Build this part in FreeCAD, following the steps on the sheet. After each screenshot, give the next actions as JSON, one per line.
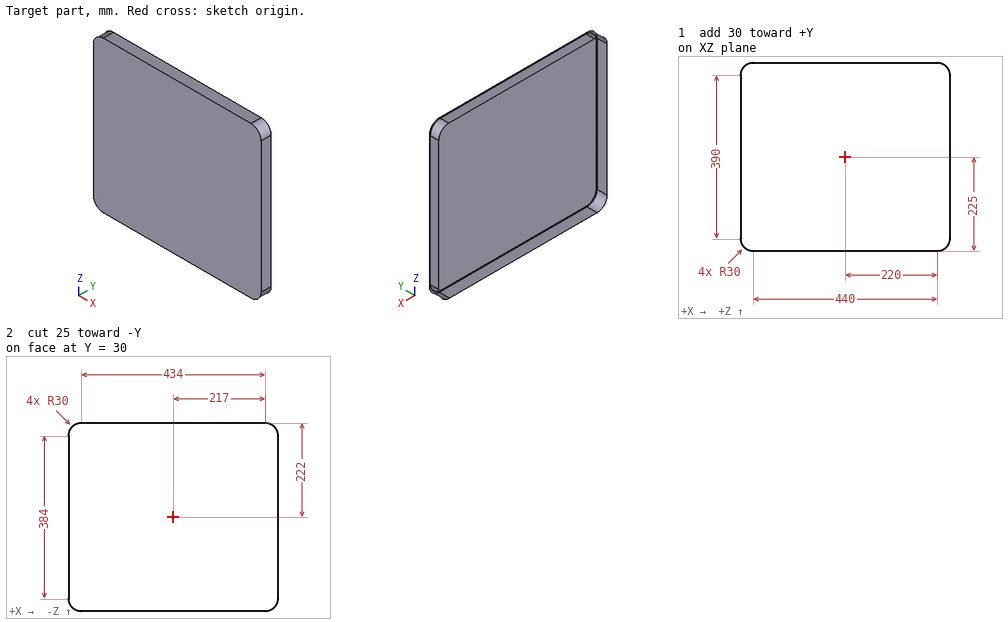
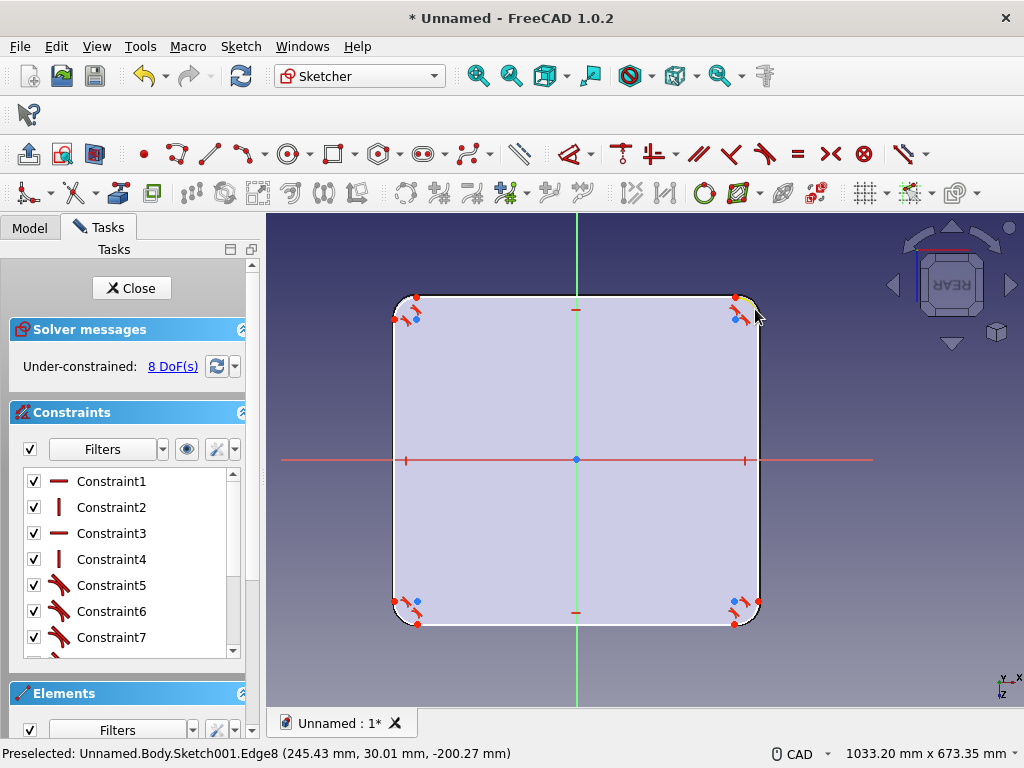
{"action": "scroll", "coordinate": [407, 300], "scroll_direction": "up", "scroll_amount": 2}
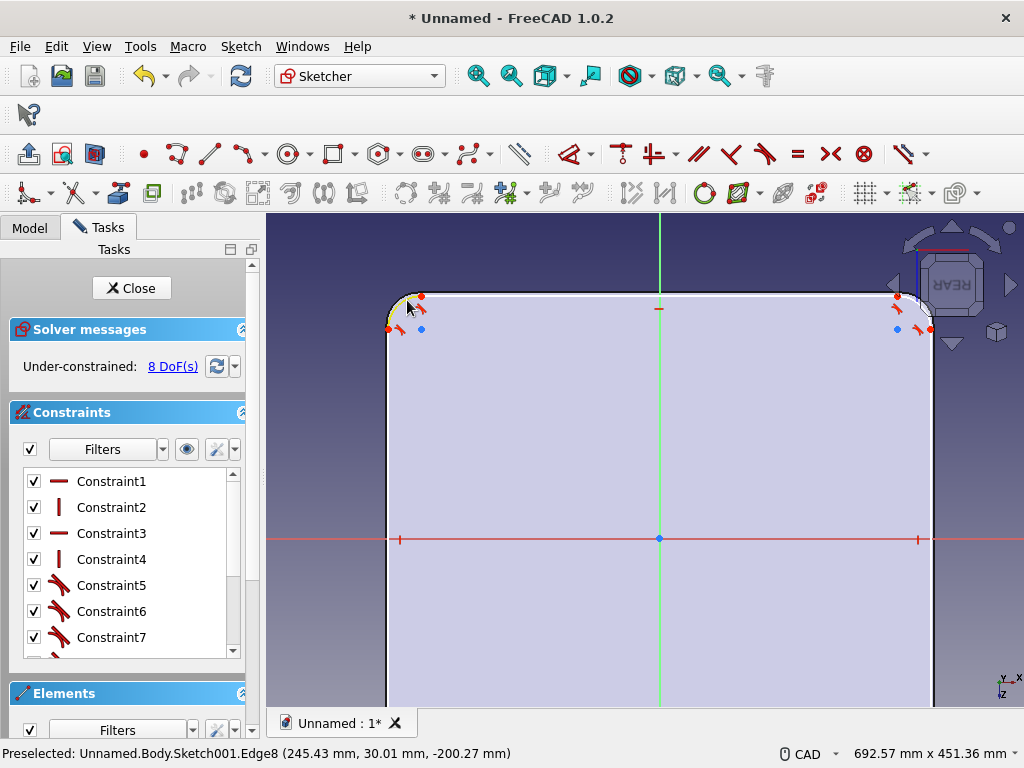
{"action": "left_click", "coordinate": [406, 300]}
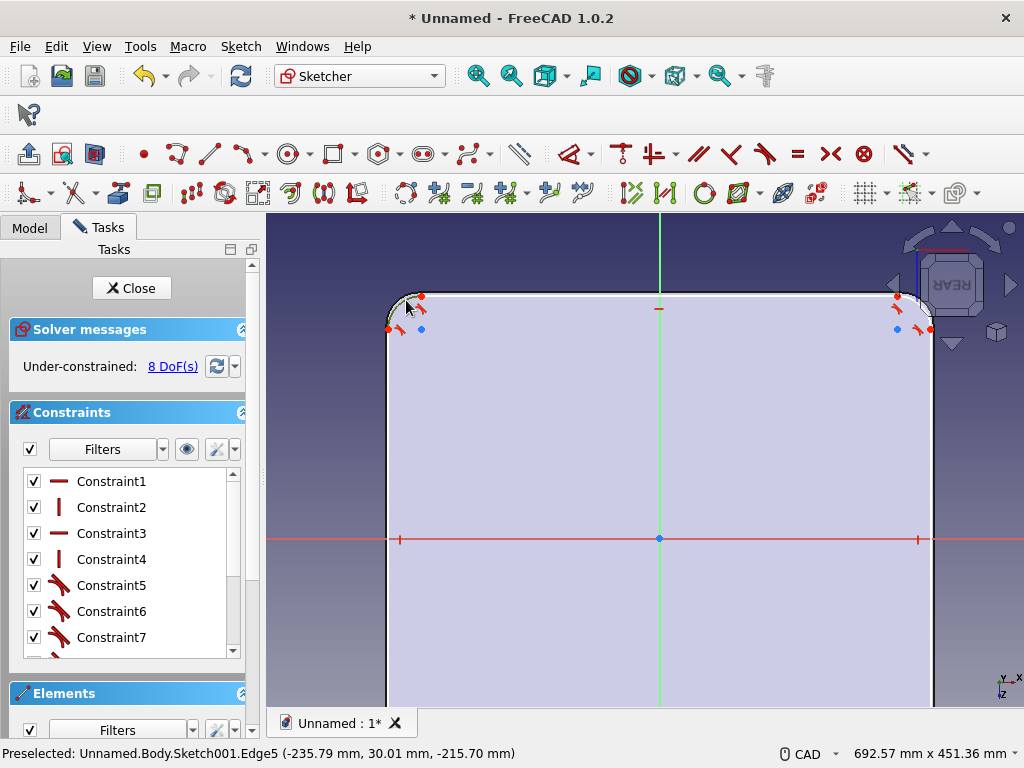
{"action": "scroll", "coordinate": [407, 300], "scroll_direction": "down", "scroll_amount": 2}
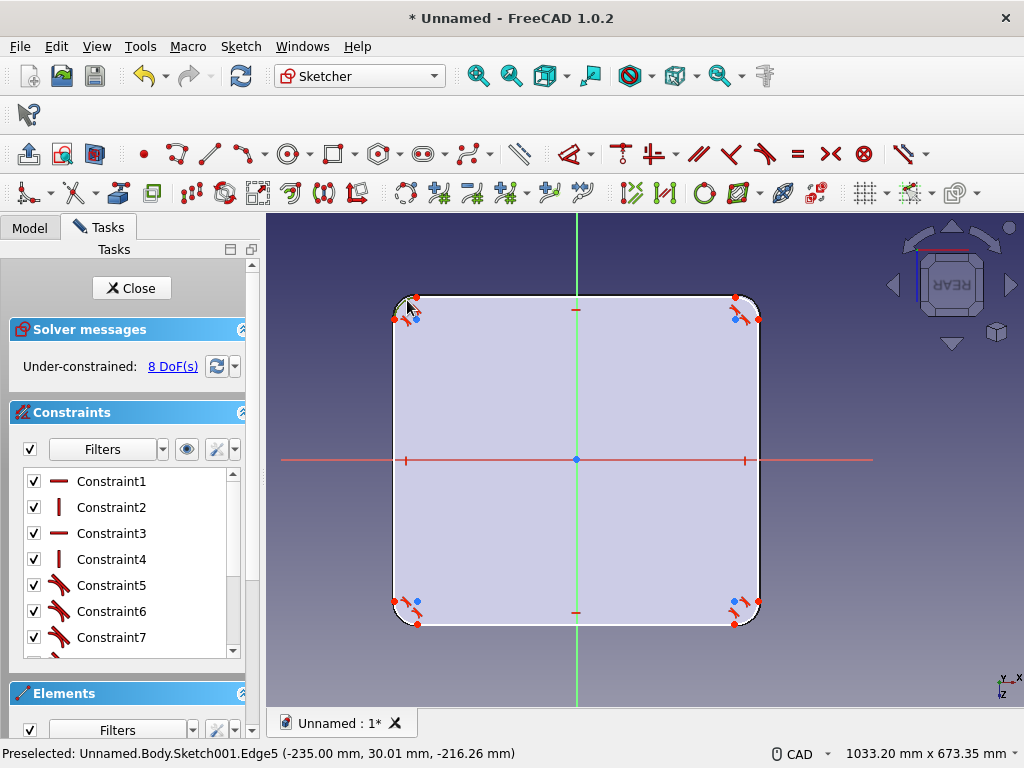
{"action": "scroll", "coordinate": [397, 612], "scroll_direction": "up", "scroll_amount": 2}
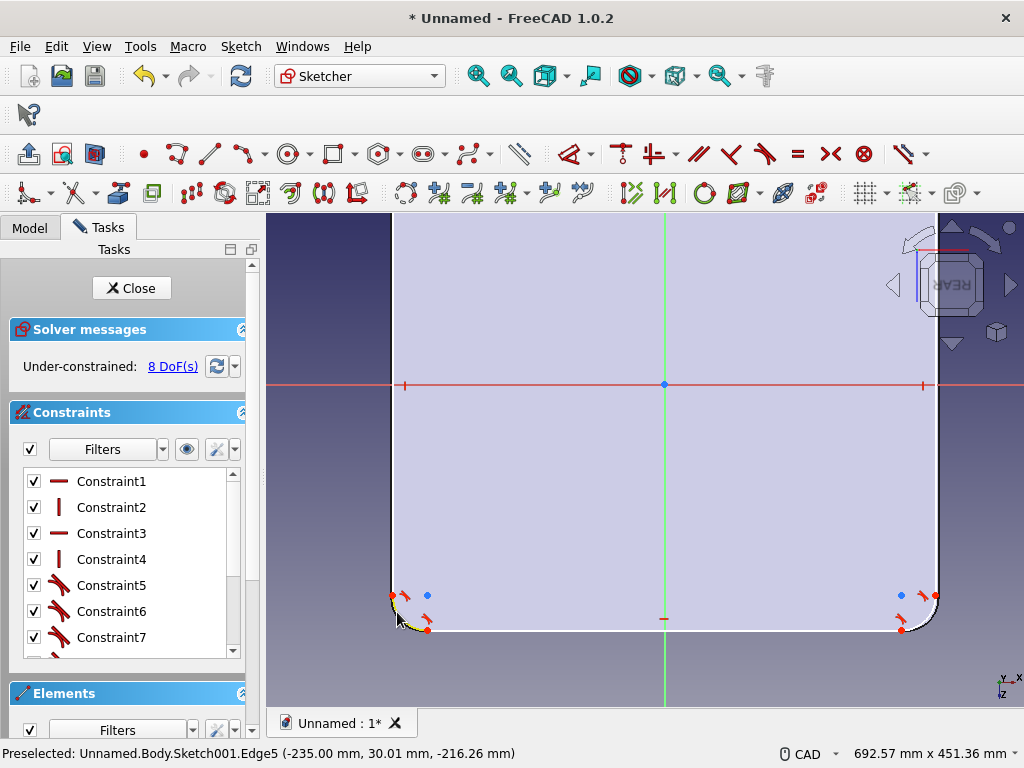
{"action": "left_click", "coordinate": [397, 612]}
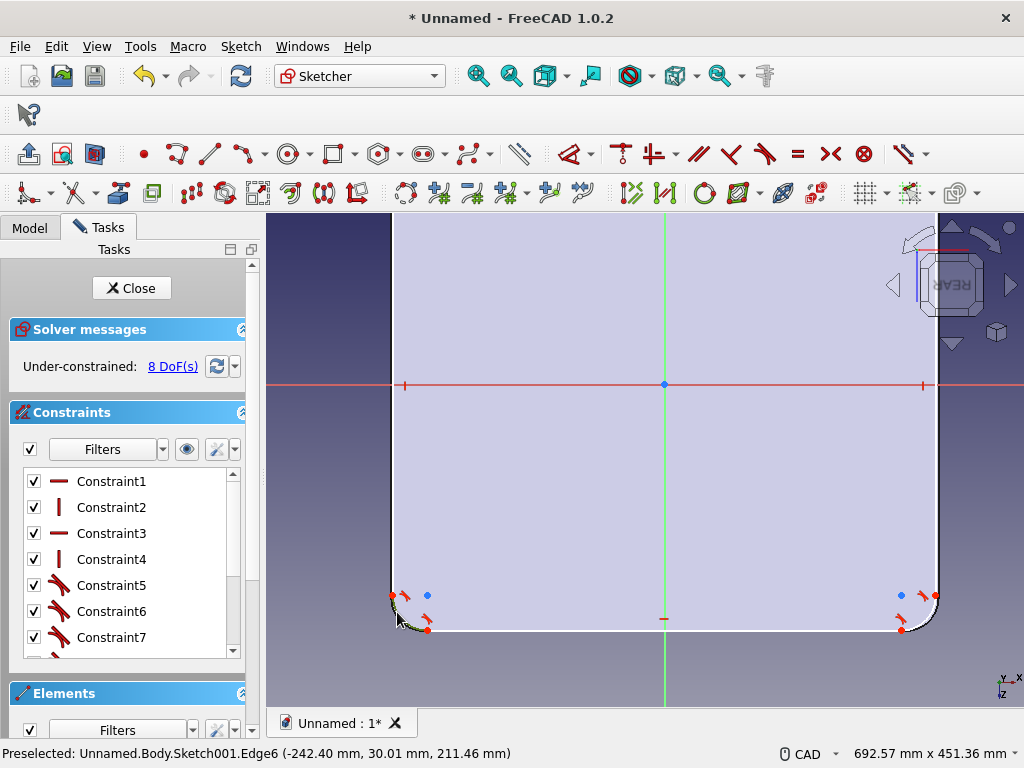
{"action": "scroll", "coordinate": [397, 613], "scroll_direction": "down", "scroll_amount": 2}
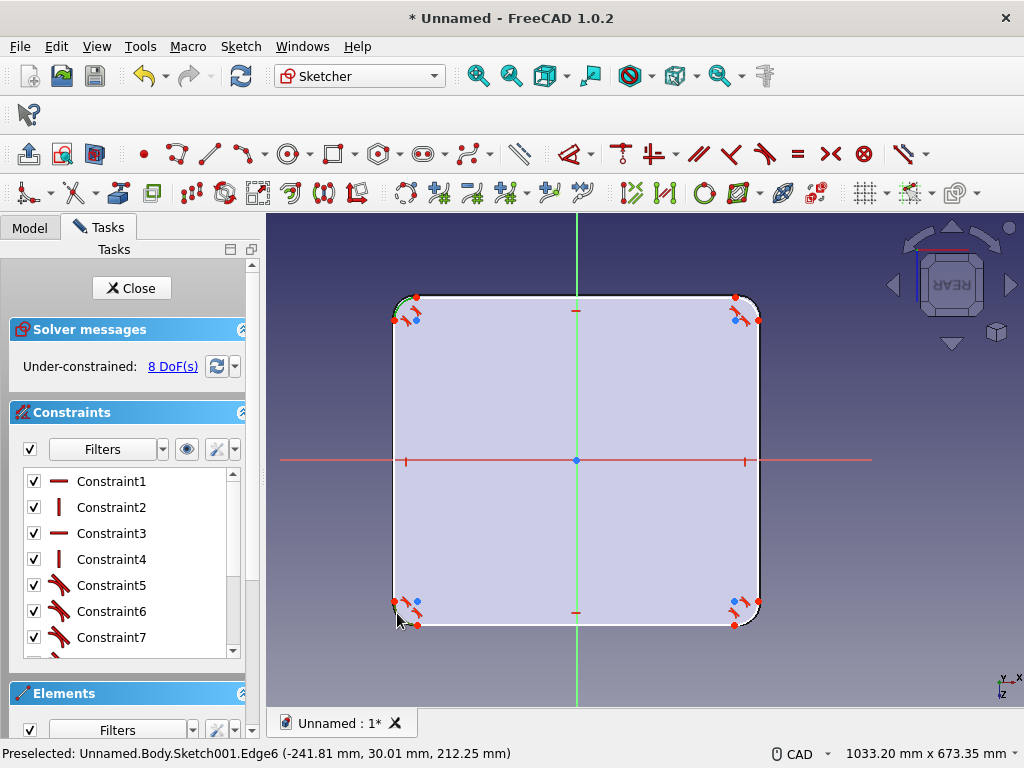
{"action": "scroll", "coordinate": [746, 623], "scroll_direction": "up", "scroll_amount": 2}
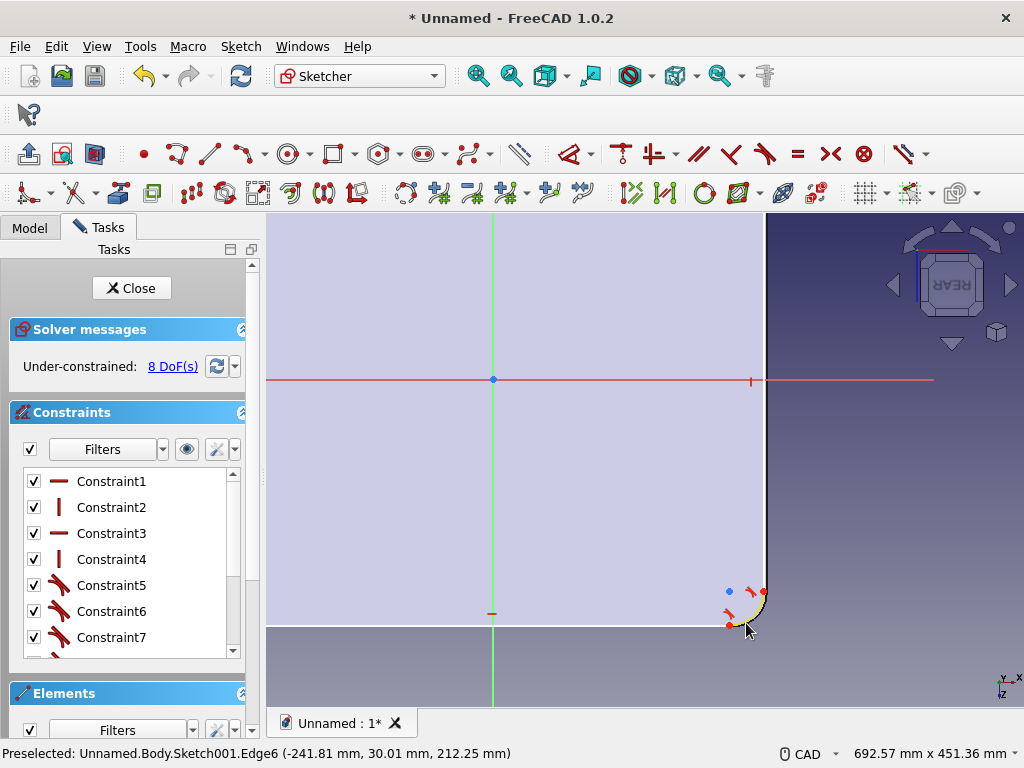
{"action": "left_click", "coordinate": [745, 622]}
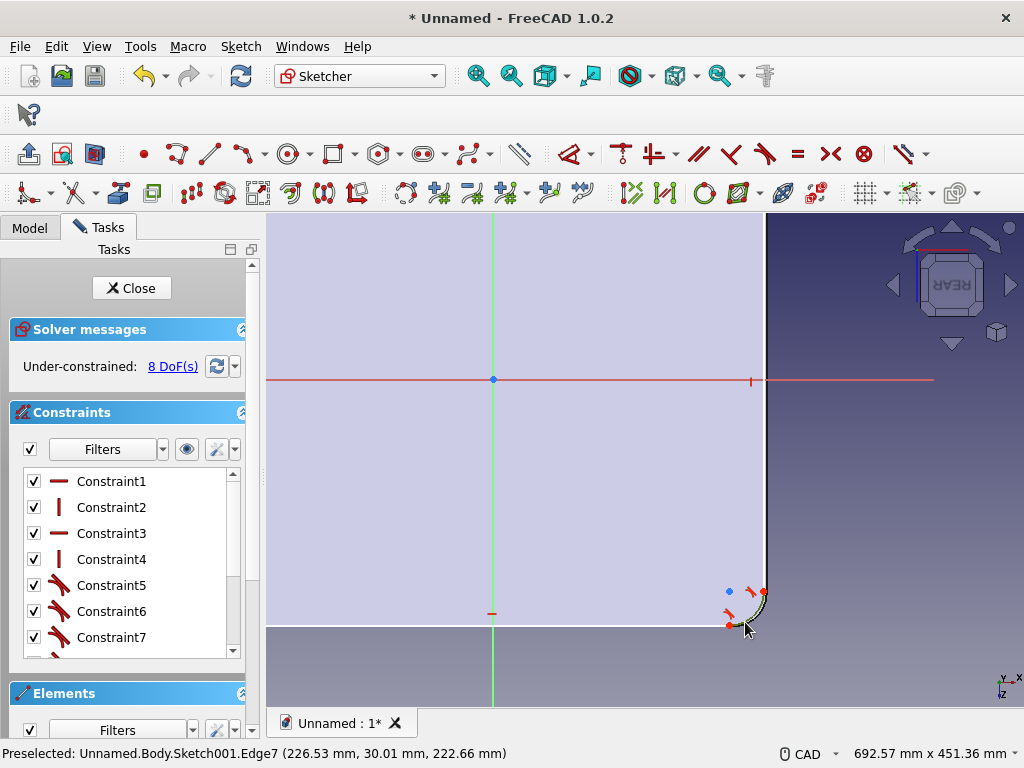
{"action": "scroll", "coordinate": [746, 623], "scroll_direction": "down", "scroll_amount": 2}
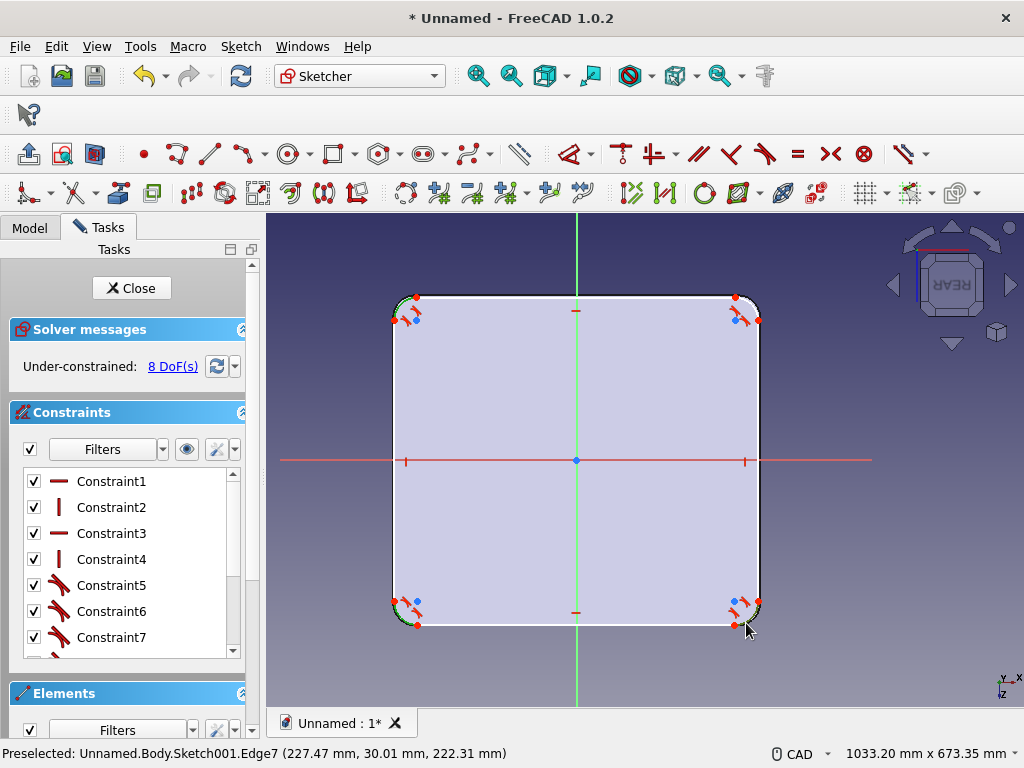
{"action": "scroll", "coordinate": [756, 310], "scroll_direction": "up", "scroll_amount": 2}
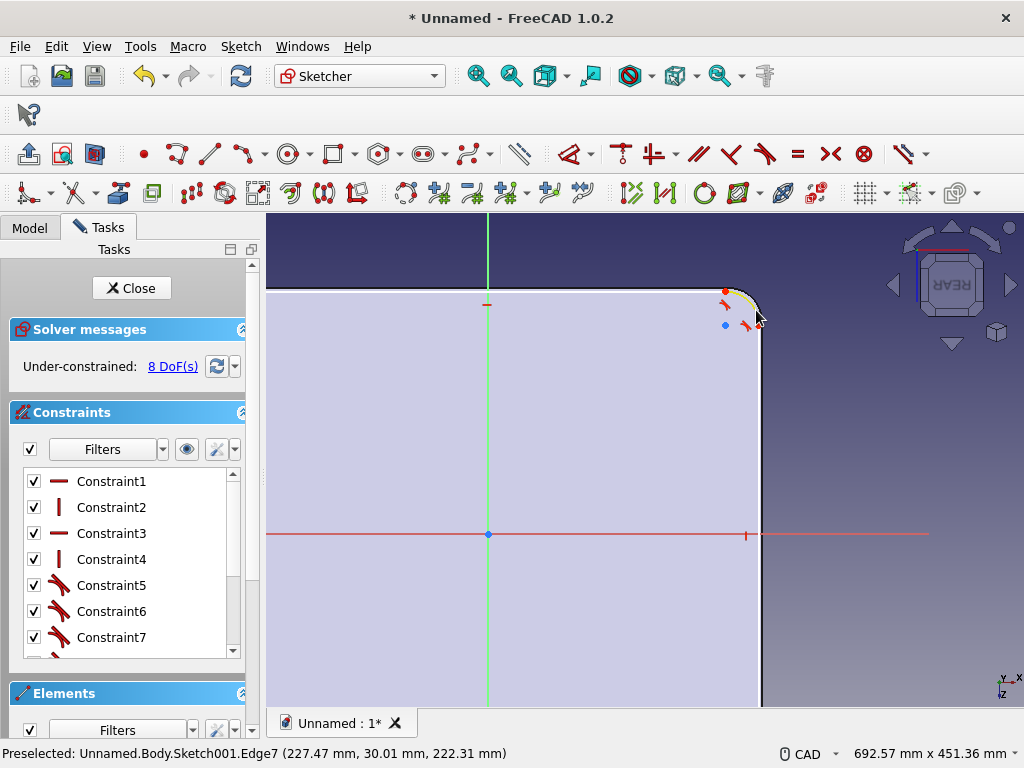
{"action": "left_click", "coordinate": [755, 310]}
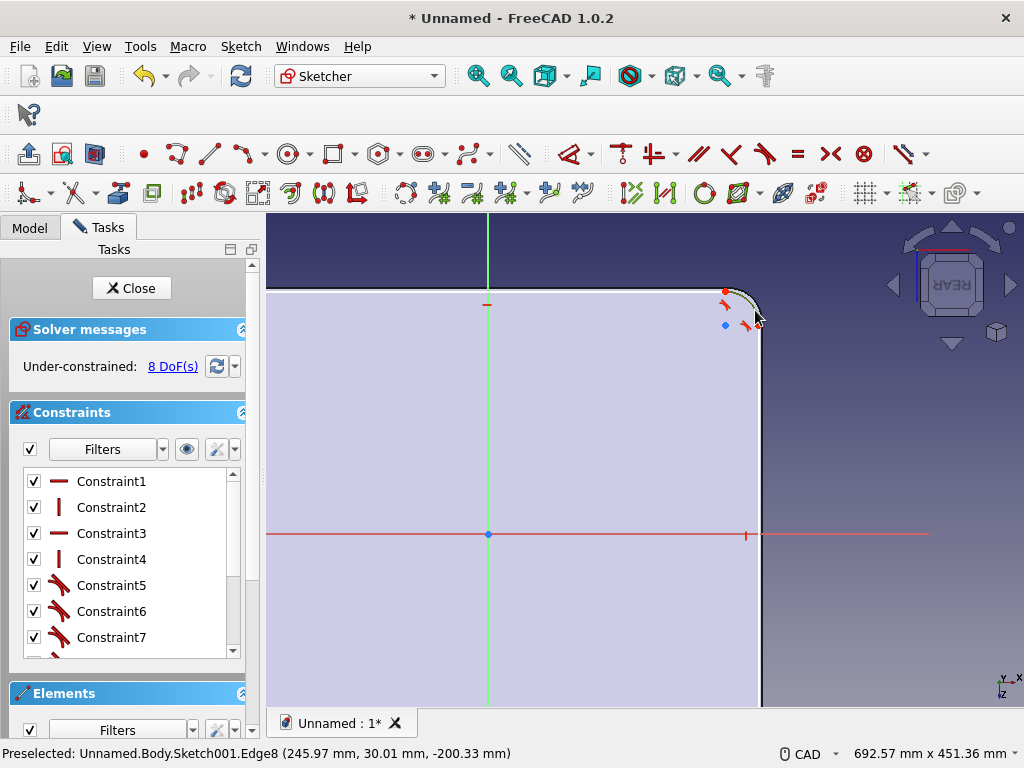
{"action": "left_click", "coordinate": [798, 154]}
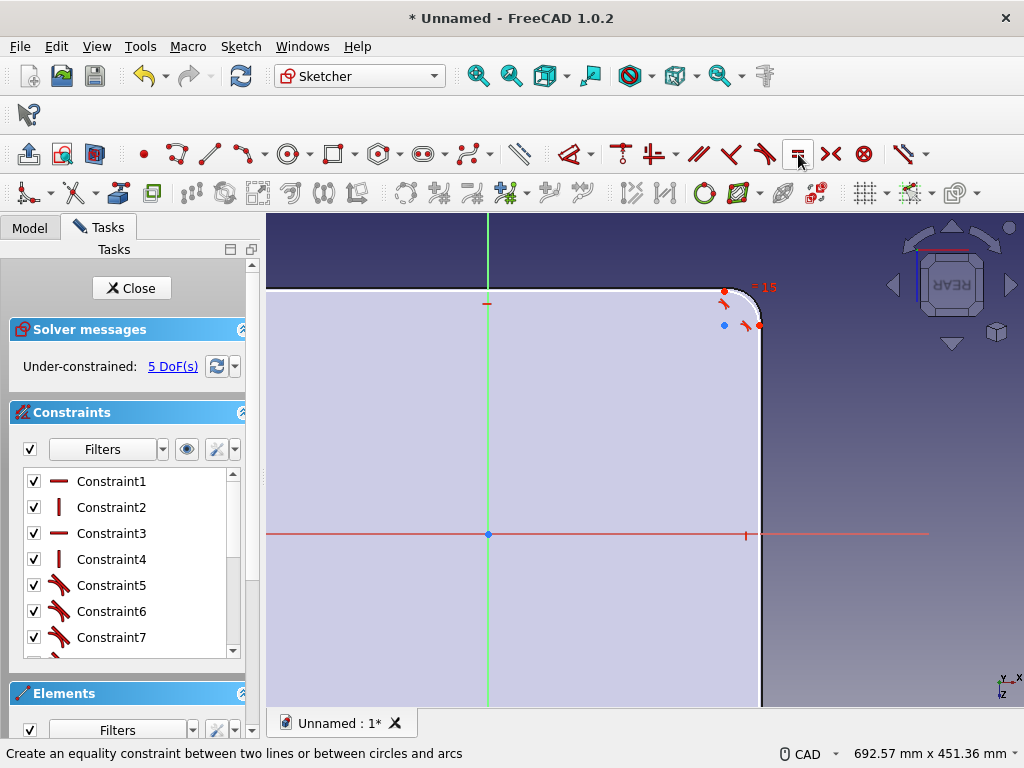
{"action": "left_click", "coordinate": [568, 154]}